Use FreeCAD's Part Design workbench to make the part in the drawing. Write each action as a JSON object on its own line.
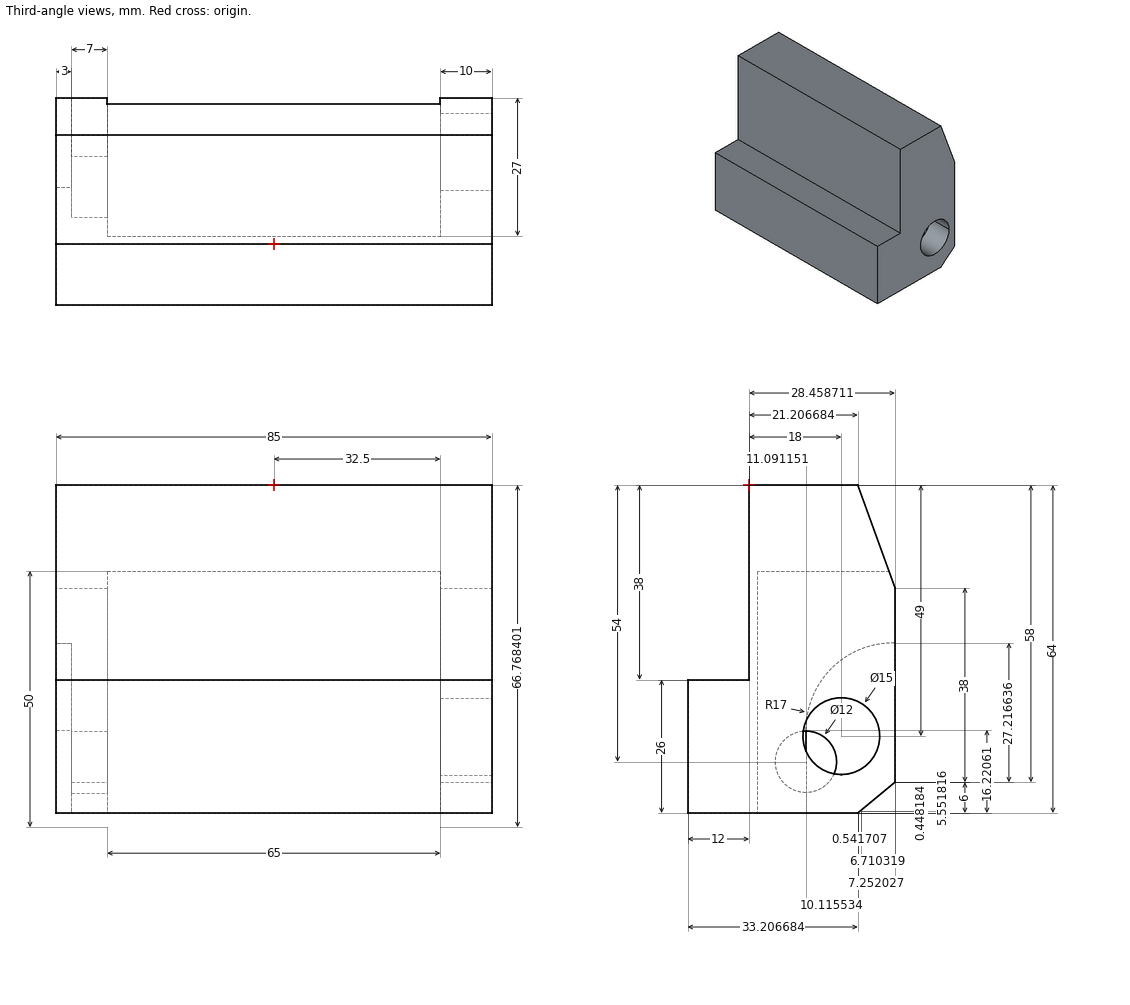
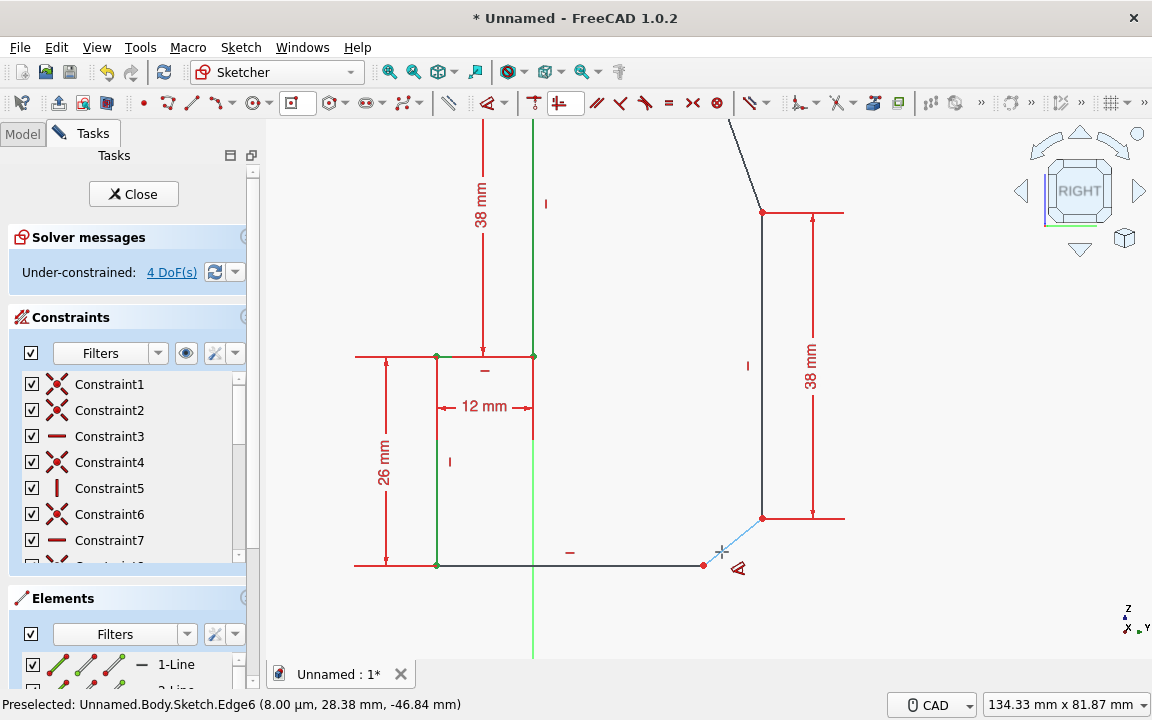
{"action": "left_click", "coordinate": [721, 552]}
{"action": "left_click", "coordinate": [796, 542]}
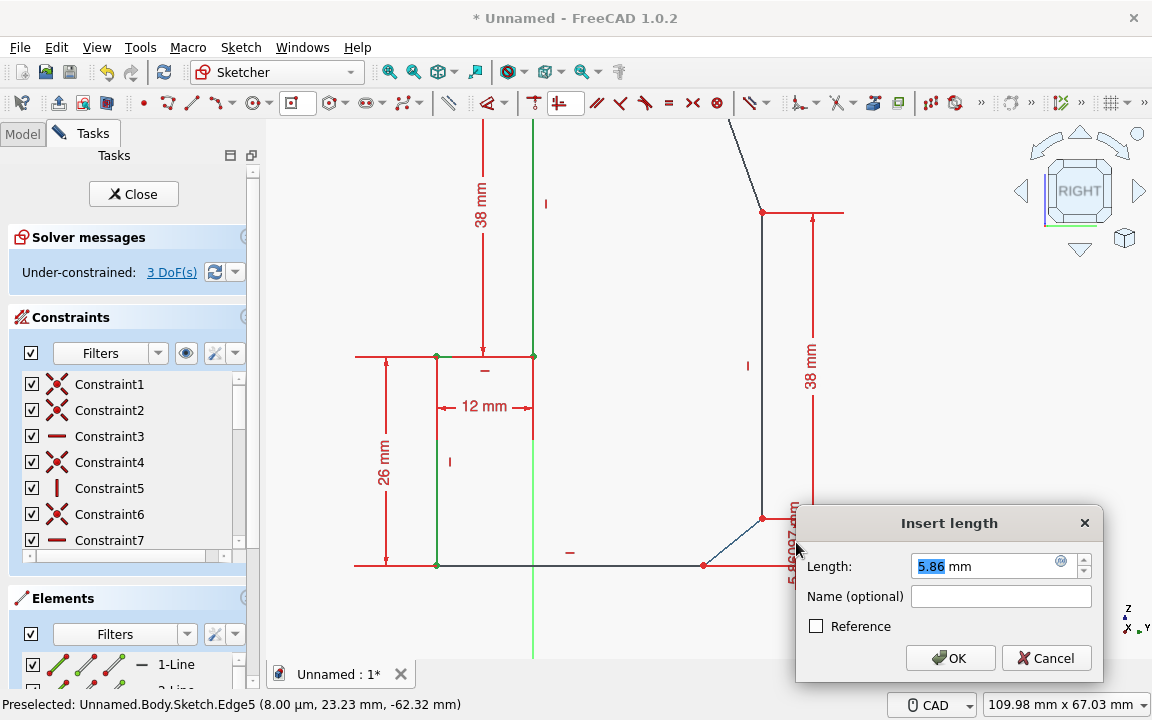
{"action": "type", "text": "6"}
{"action": "key", "text": "Return"}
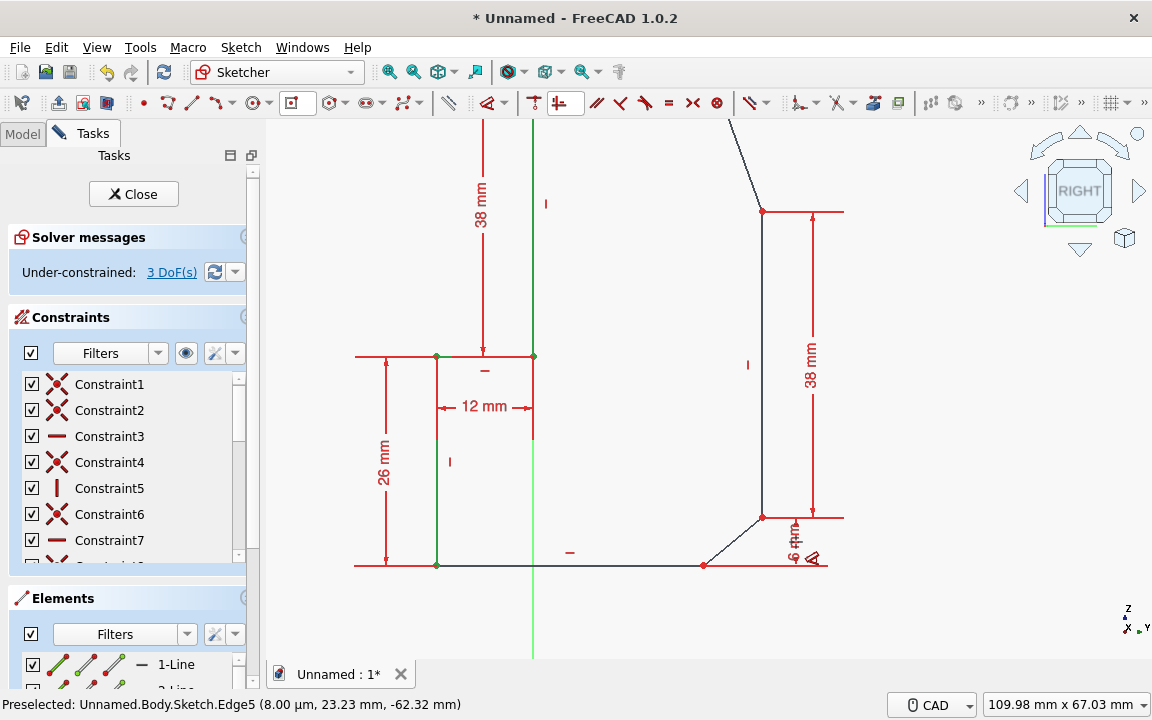
{"action": "left_click", "coordinate": [517, 566]}
{"action": "left_click", "coordinate": [570, 600]}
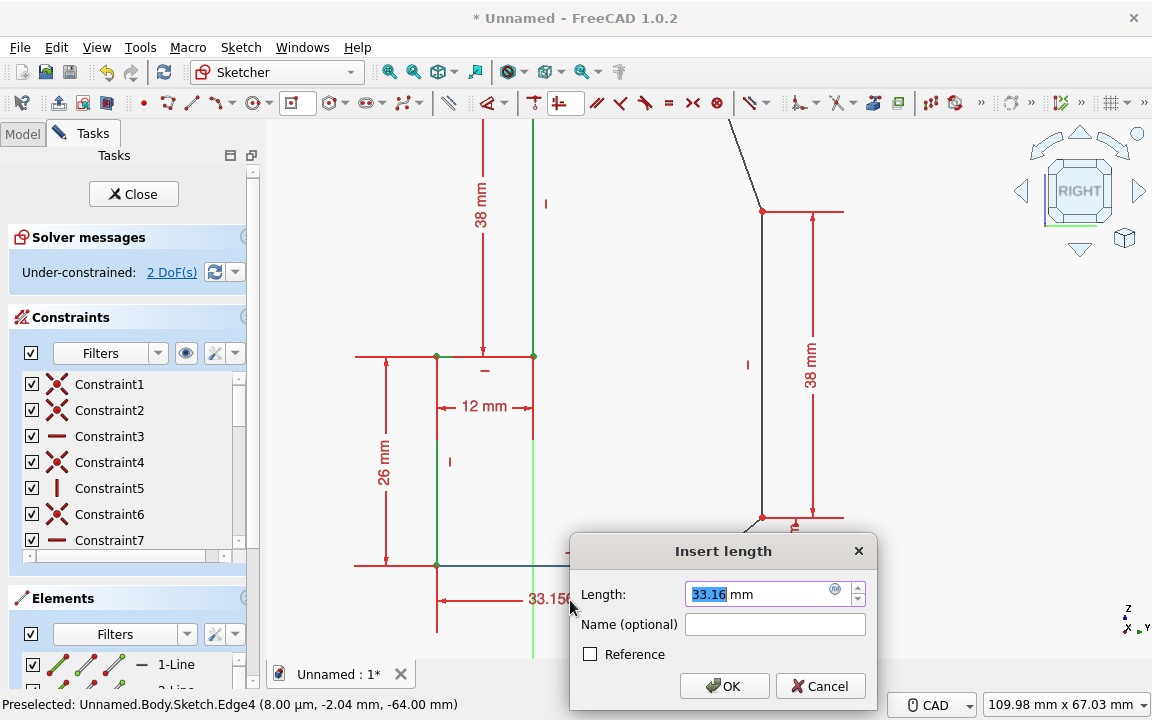
{"action": "type", "text": "33.206684"}
{"action": "key", "text": "Return"}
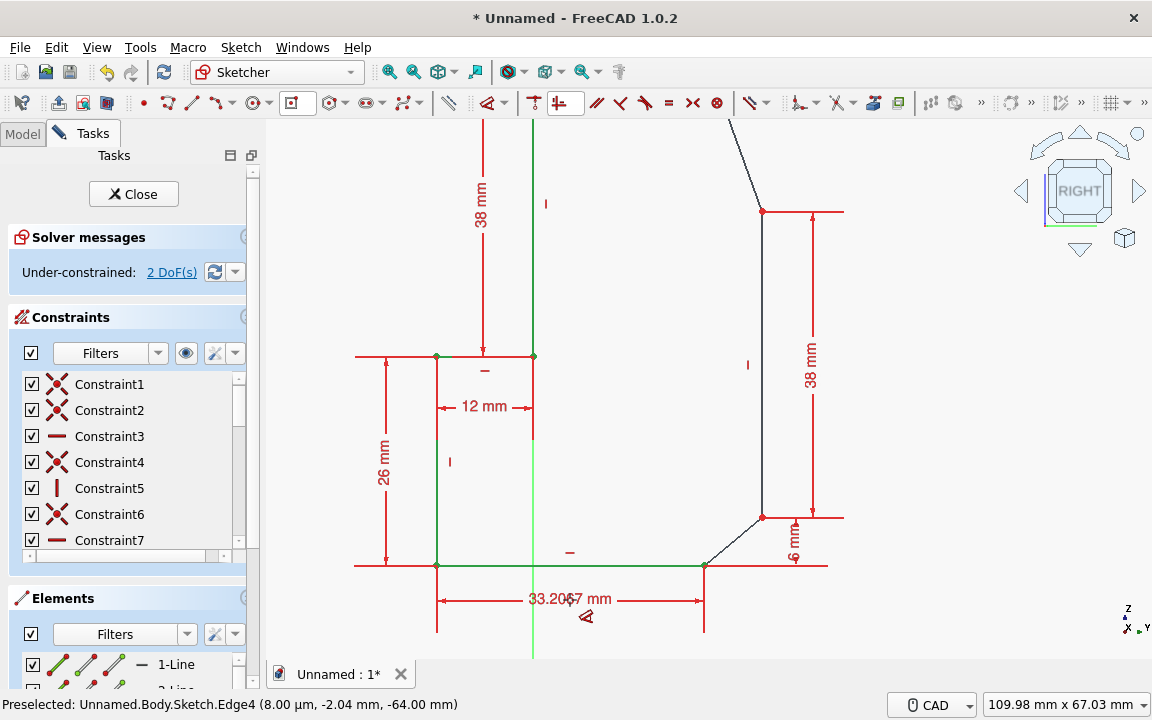
{"action": "scroll", "coordinate": [723, 553], "scroll_direction": "down", "scroll_amount": 2}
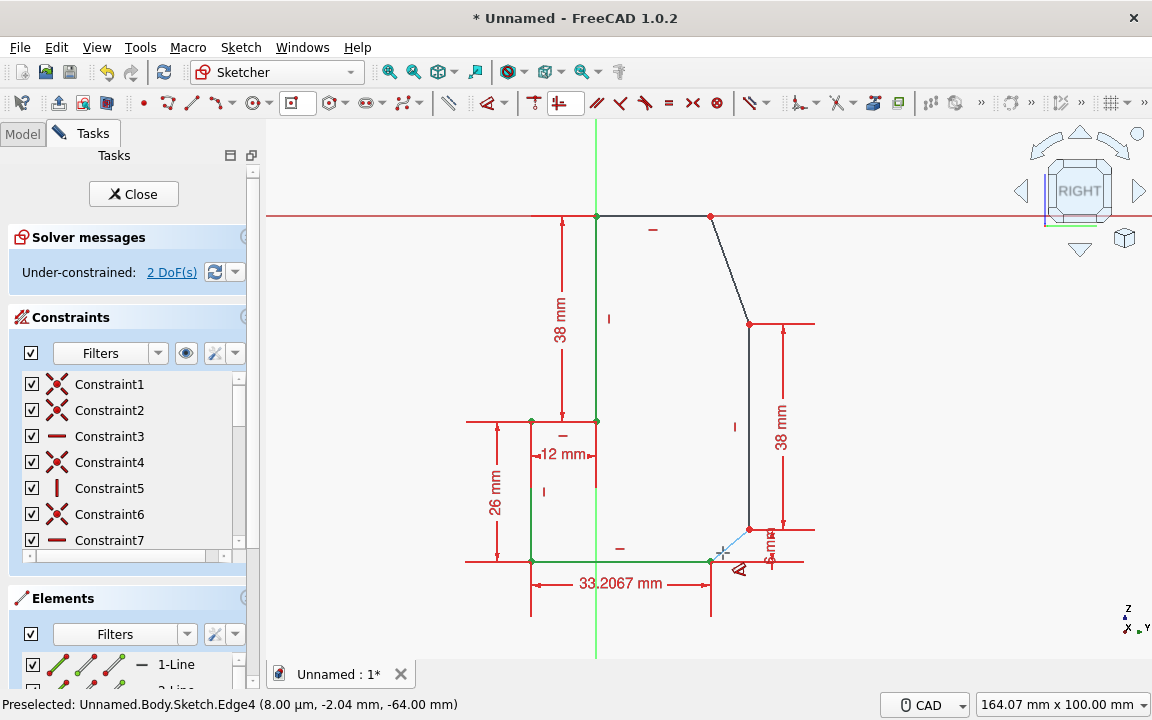
{"action": "left_click", "coordinate": [676, 216]}
{"action": "left_click", "coordinate": [653, 182]}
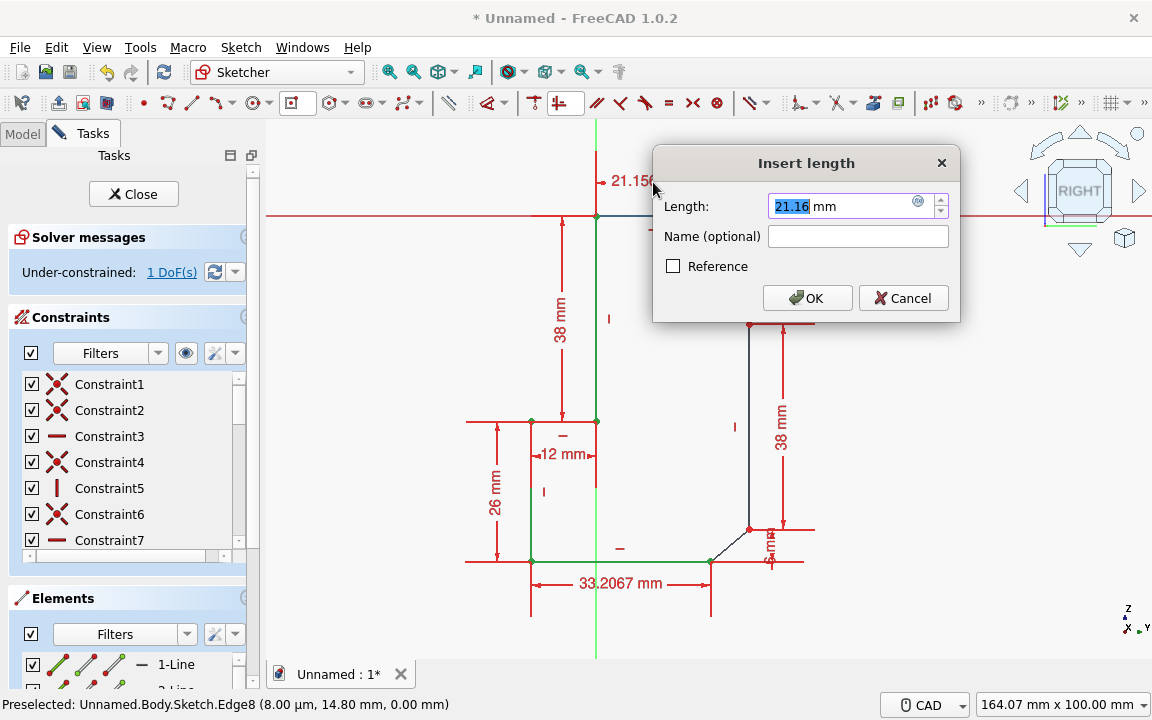
{"action": "type", "text": "21.206684"}
{"action": "key", "text": "Return"}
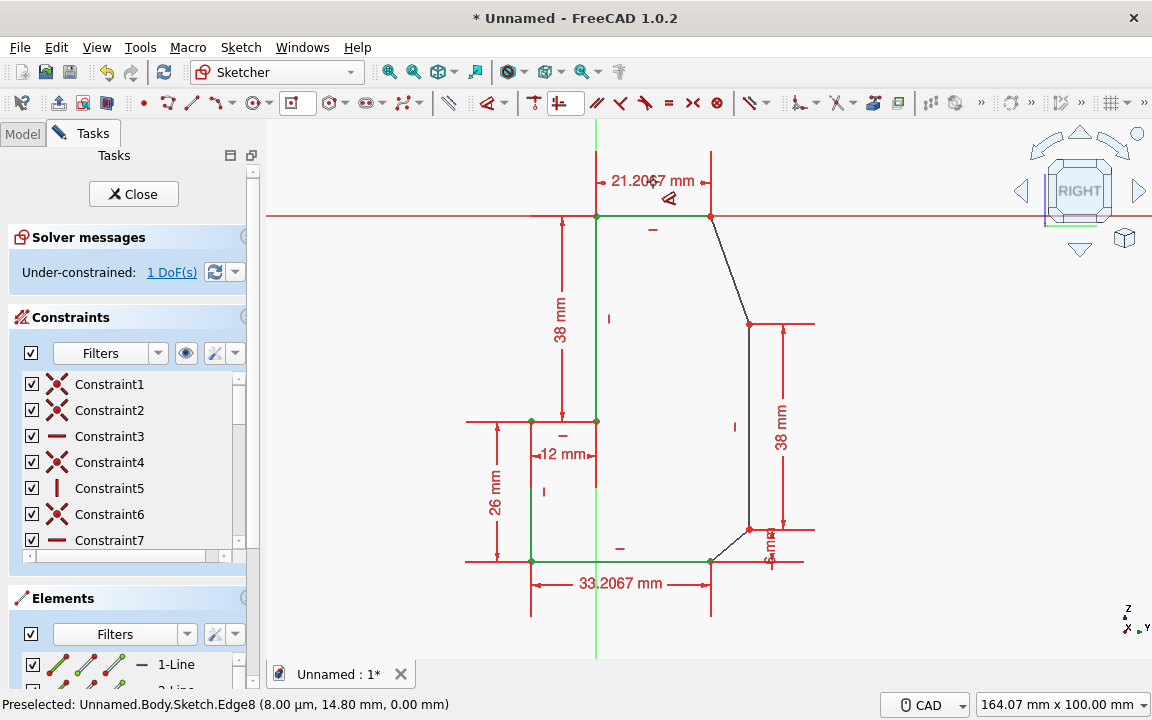
{"action": "left_click", "coordinate": [722, 552]}
{"action": "left_click", "coordinate": [730, 596]}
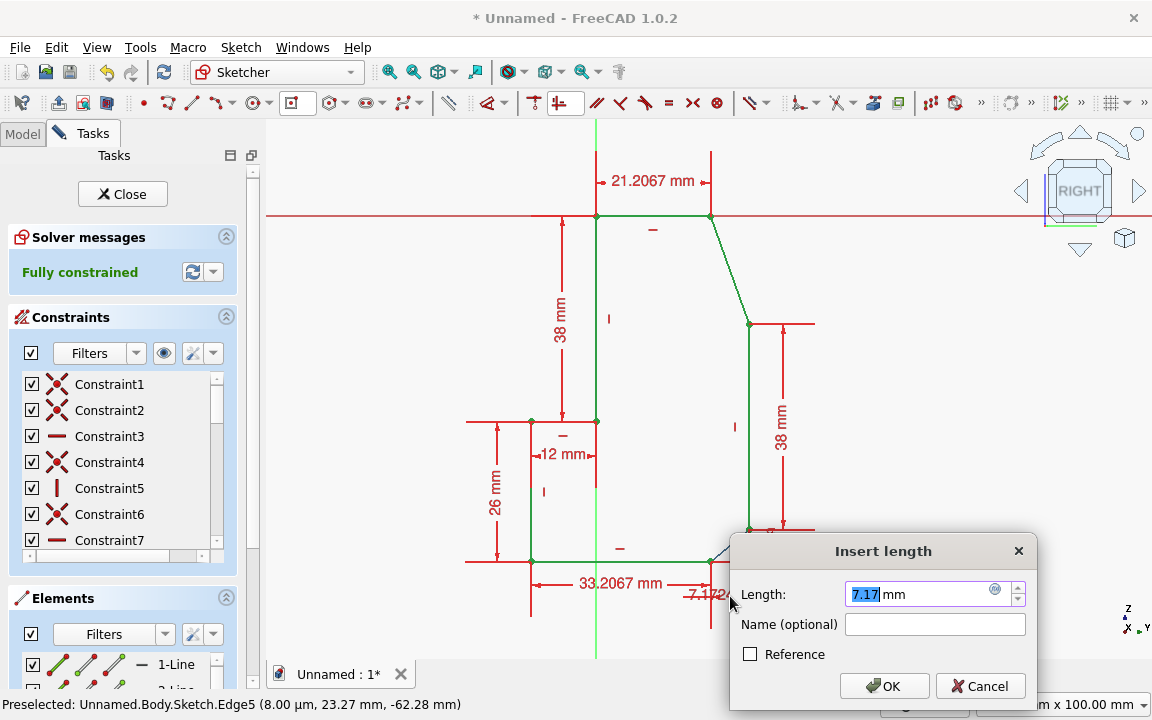
{"action": "type", "text": "7.252027"}
{"action": "key", "text": "Return"}
{"action": "key", "text": "Escape"}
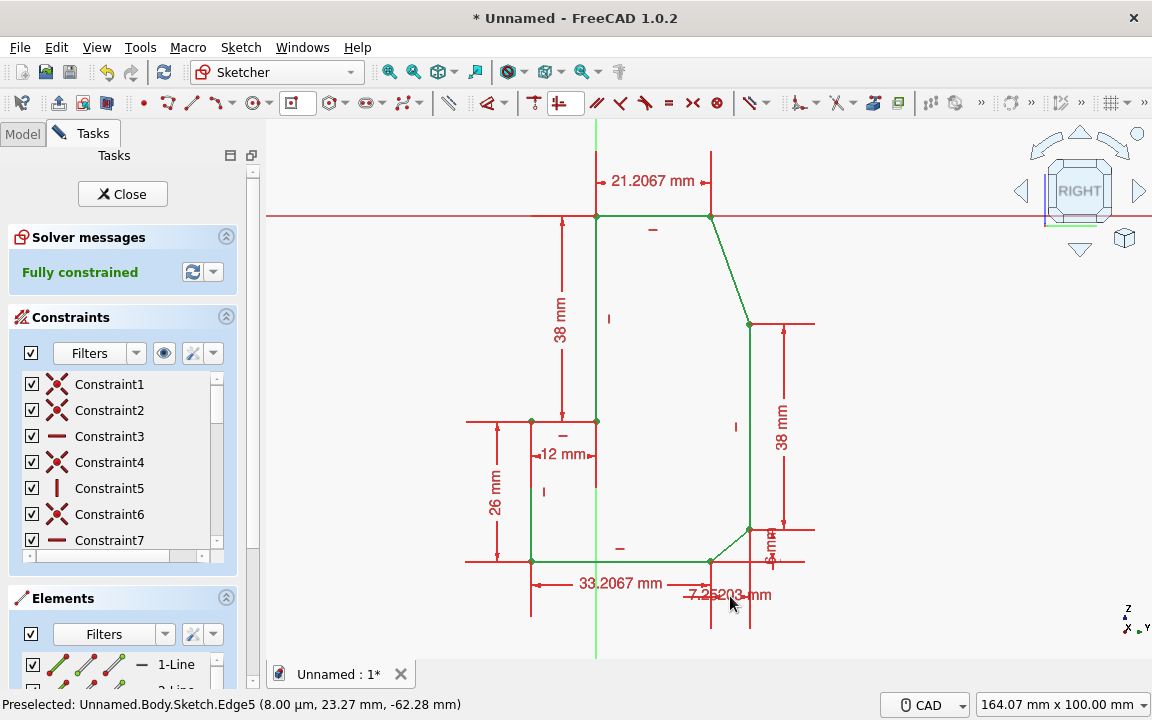
{"action": "left_click", "coordinate": [123, 194]}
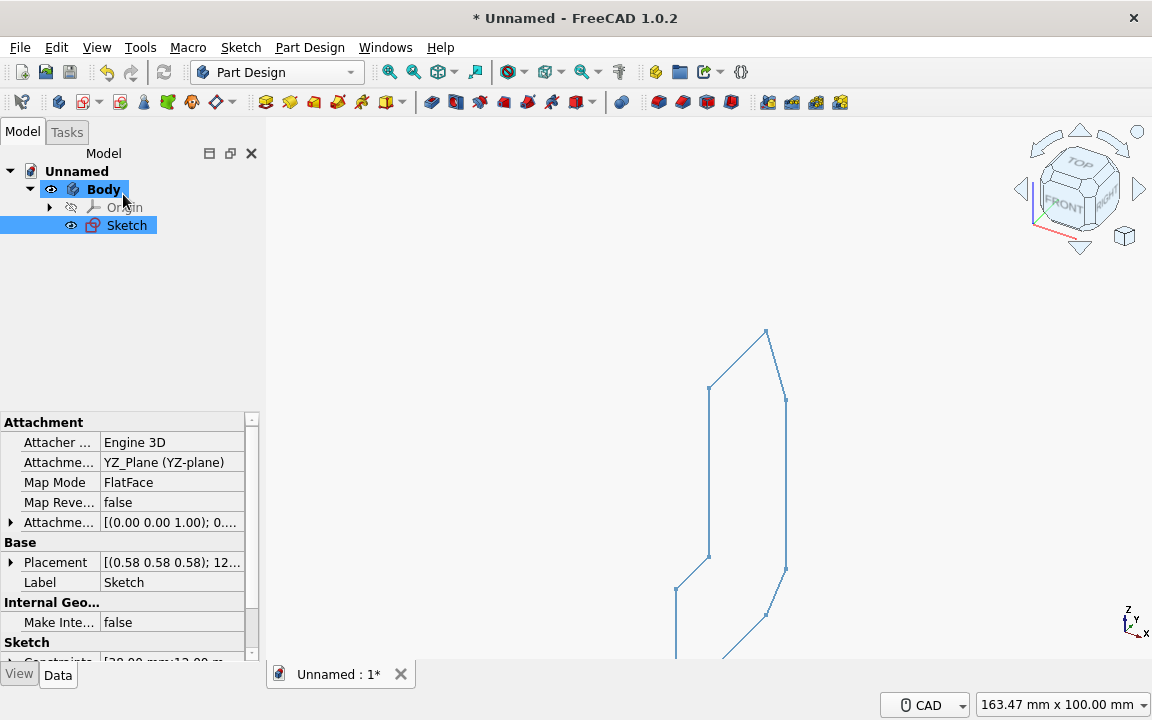
{"action": "left_click", "coordinate": [266, 102]}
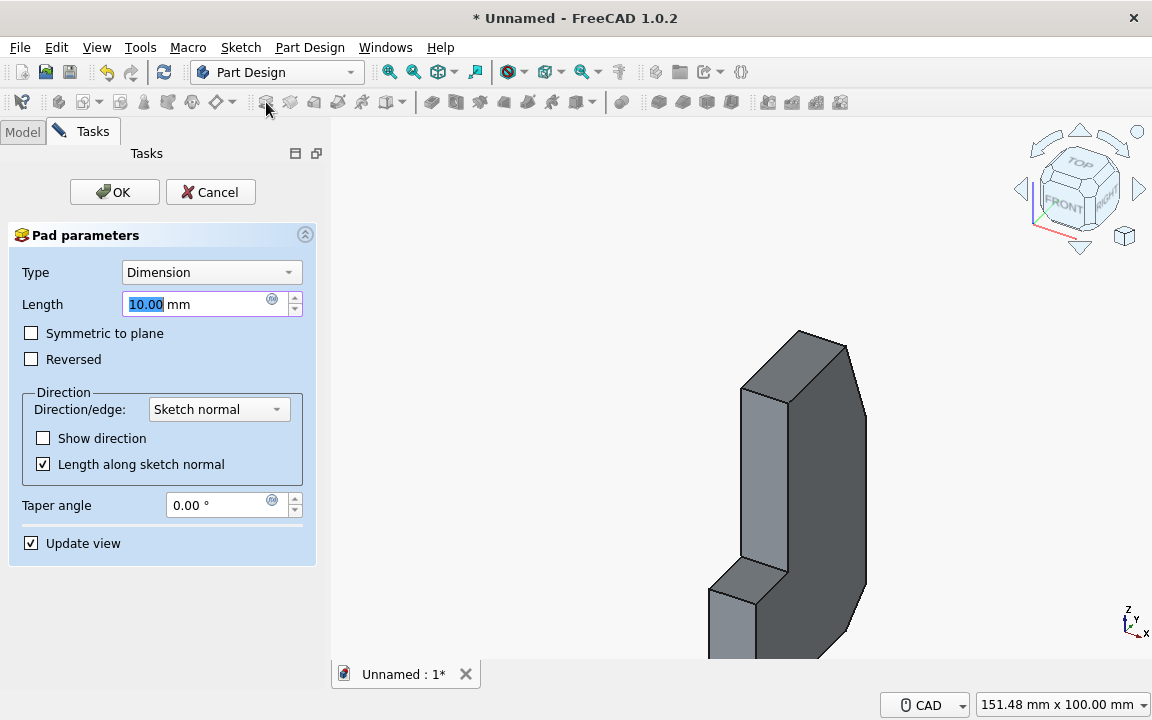
{"action": "type", "text": "85"}
{"action": "key", "text": "Tab"}